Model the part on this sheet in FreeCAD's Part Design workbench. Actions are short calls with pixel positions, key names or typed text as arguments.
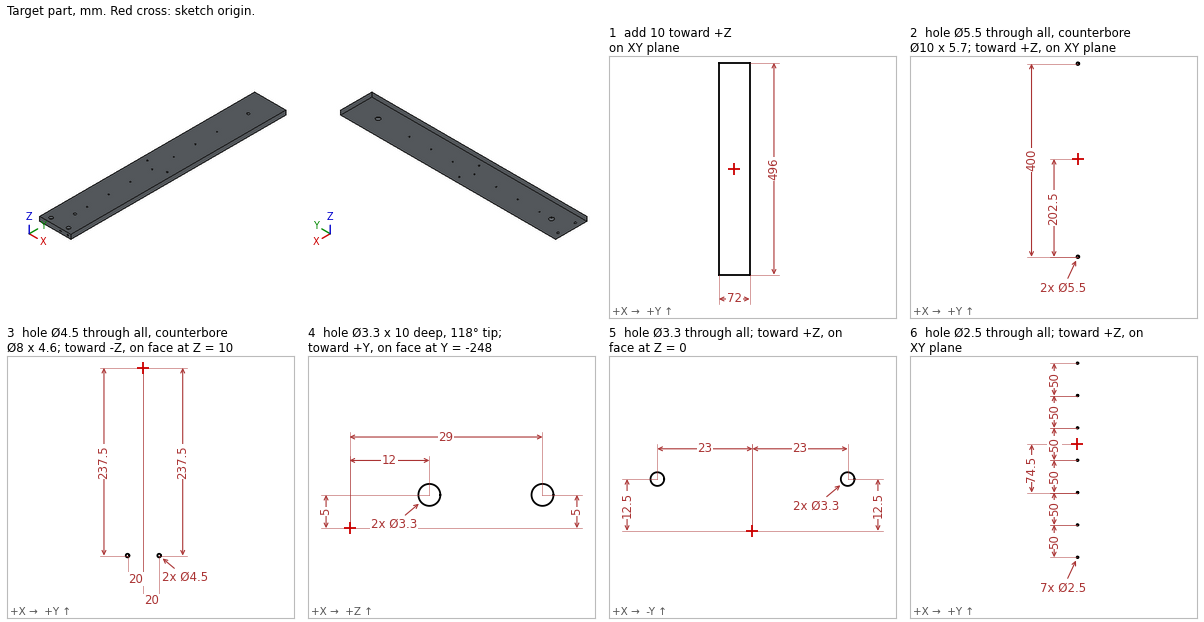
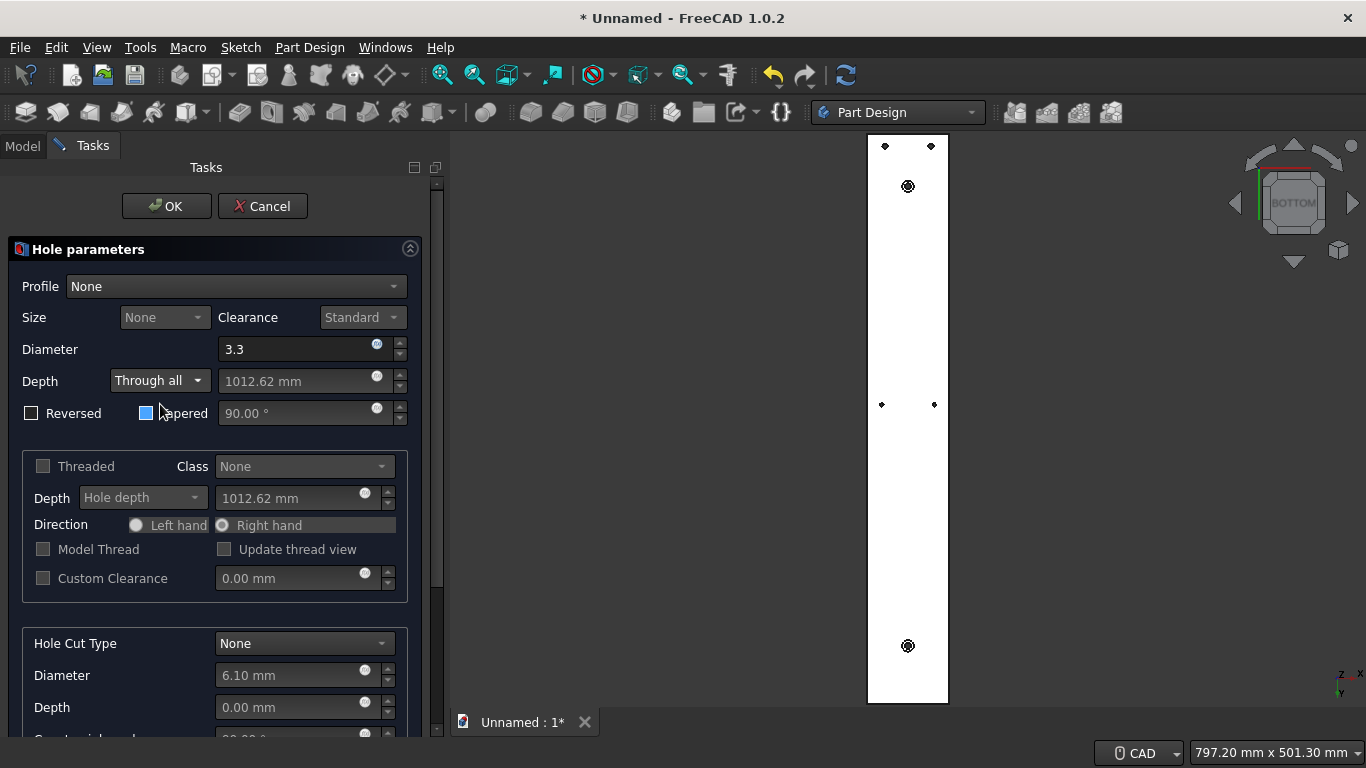
click(167, 206)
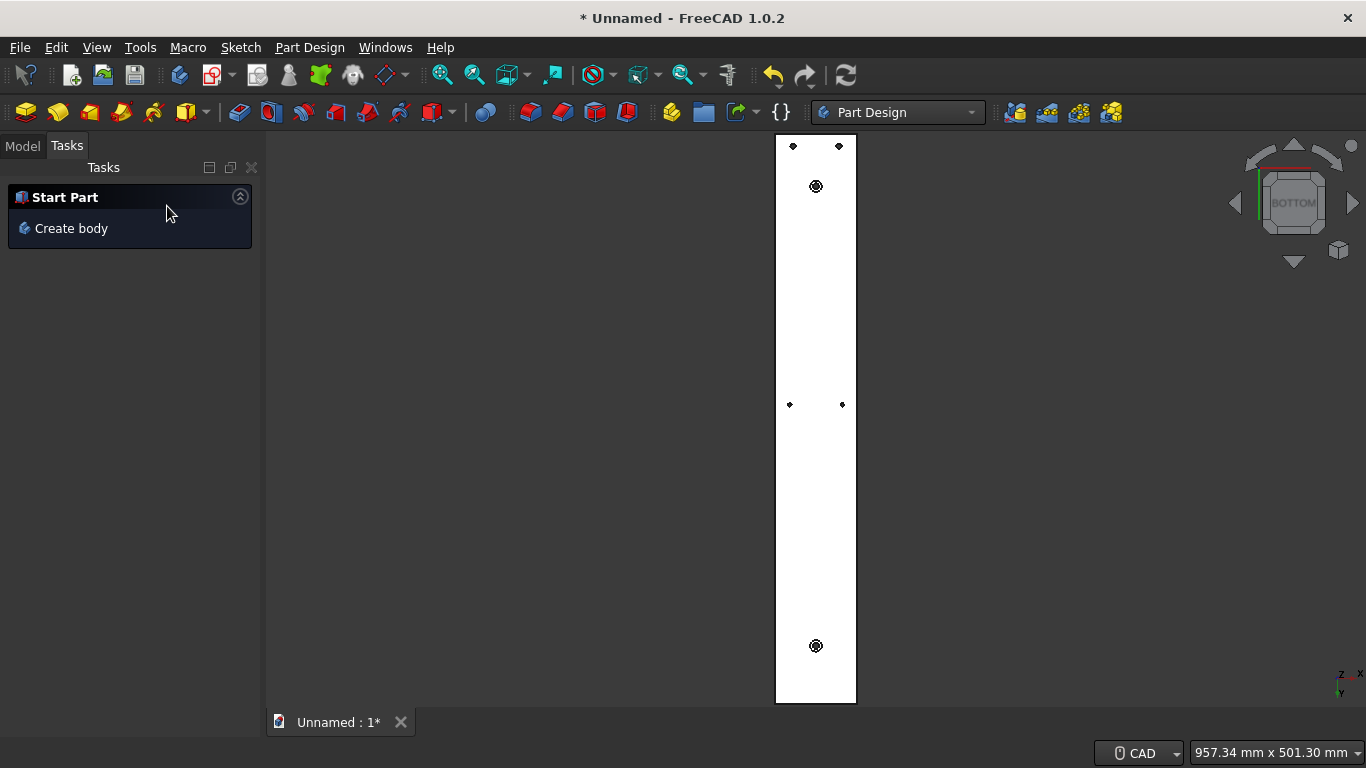
click(212, 76)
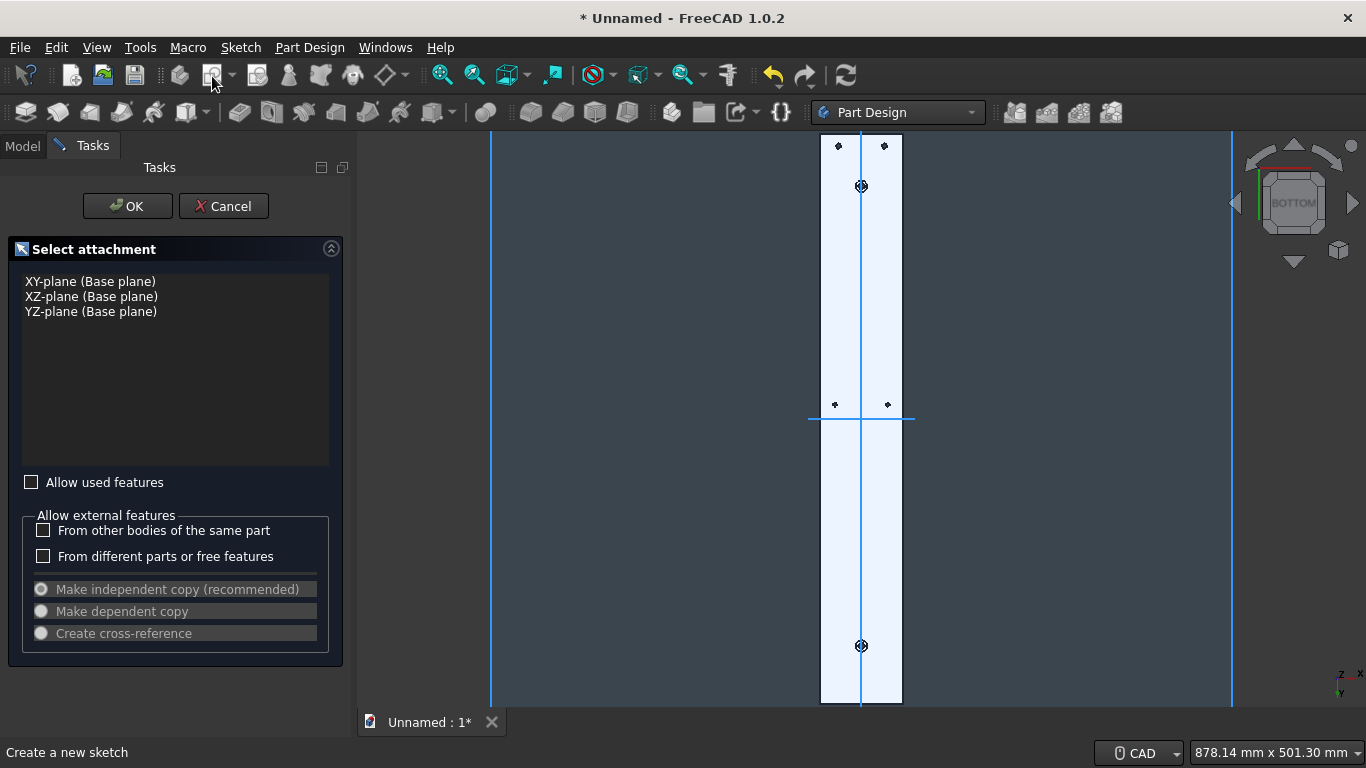
click(82, 282)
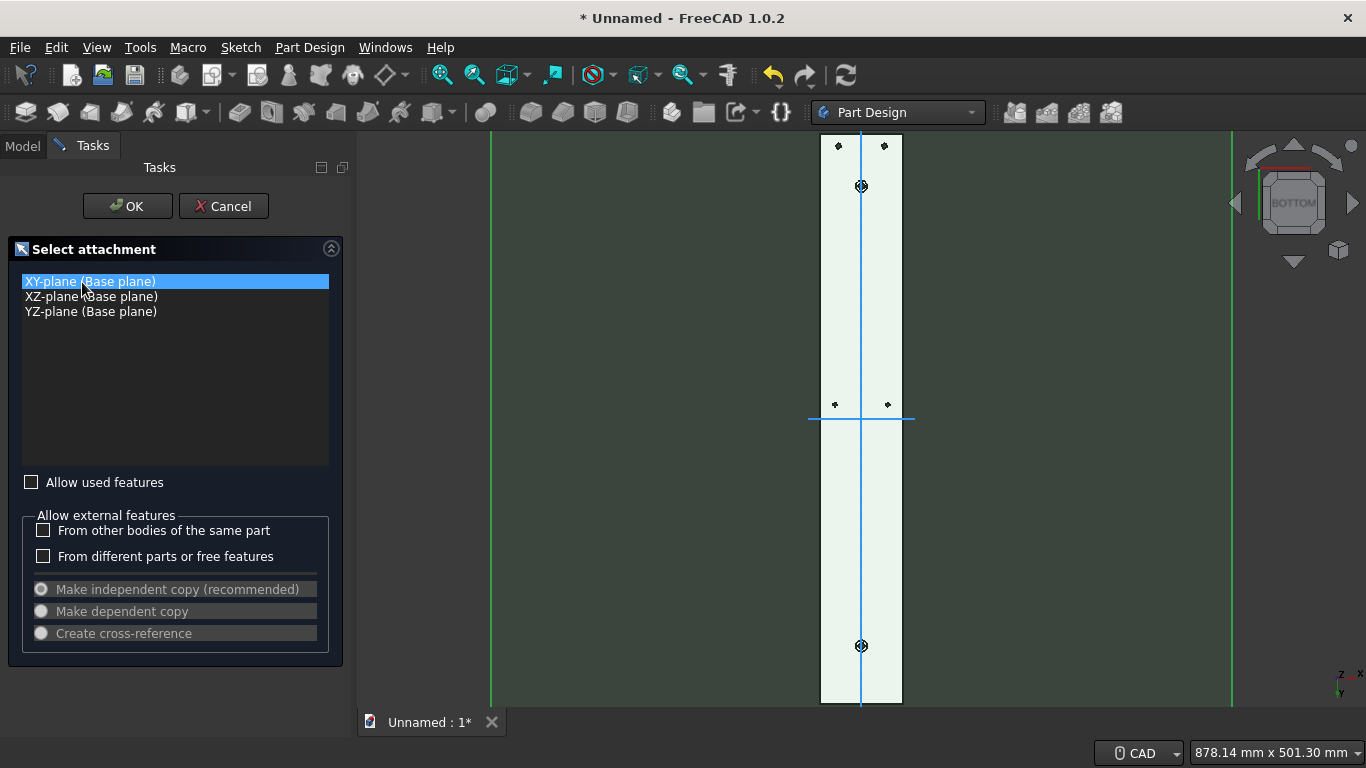
click(128, 206)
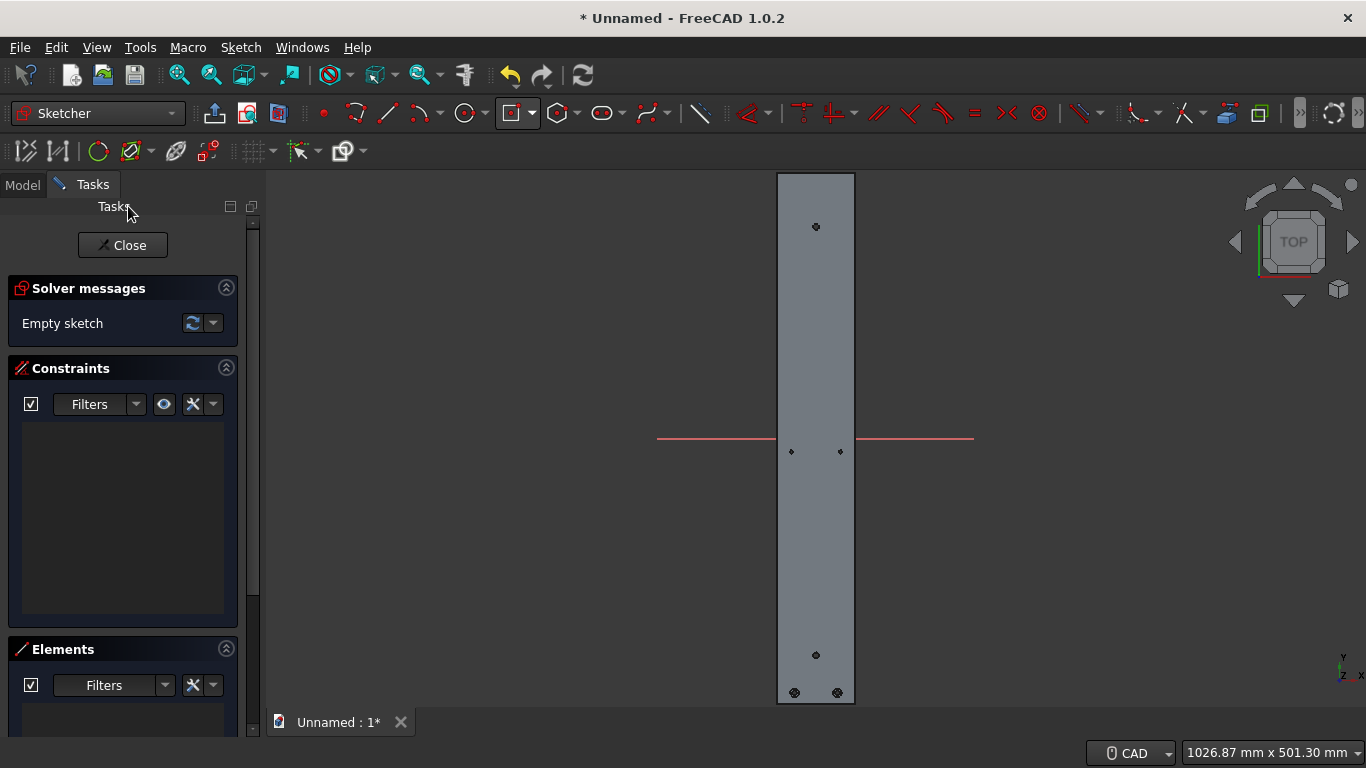
click(280, 114)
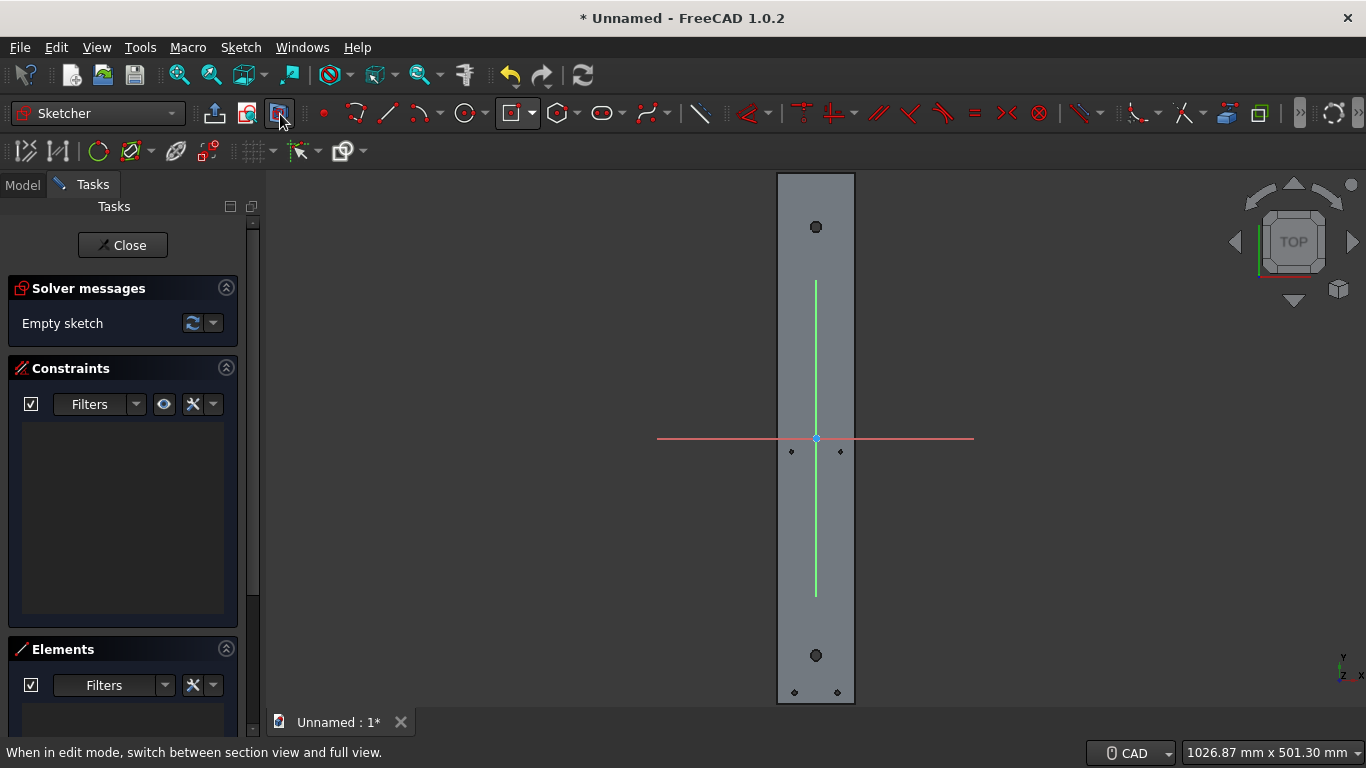
click(466, 114)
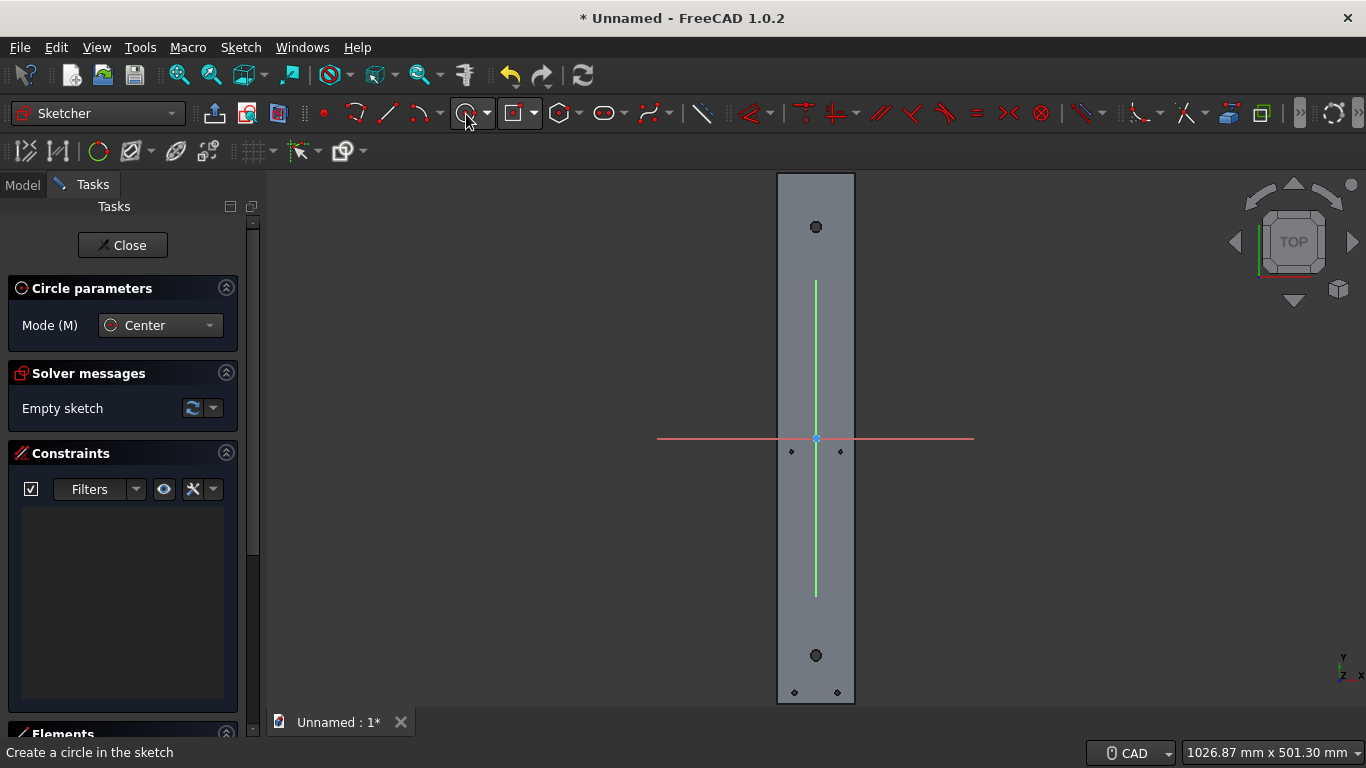
scroll(816, 625, up, 15)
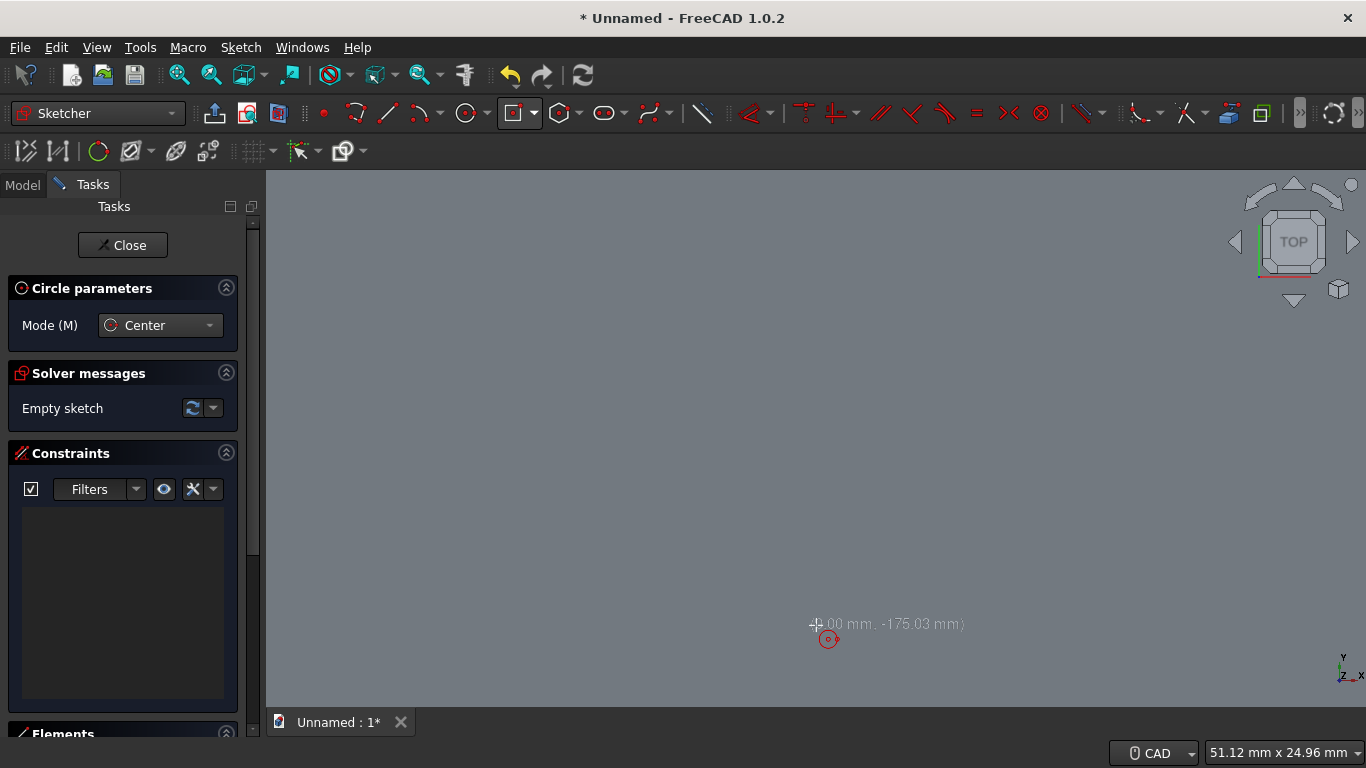
scroll(744, 598, down, 15)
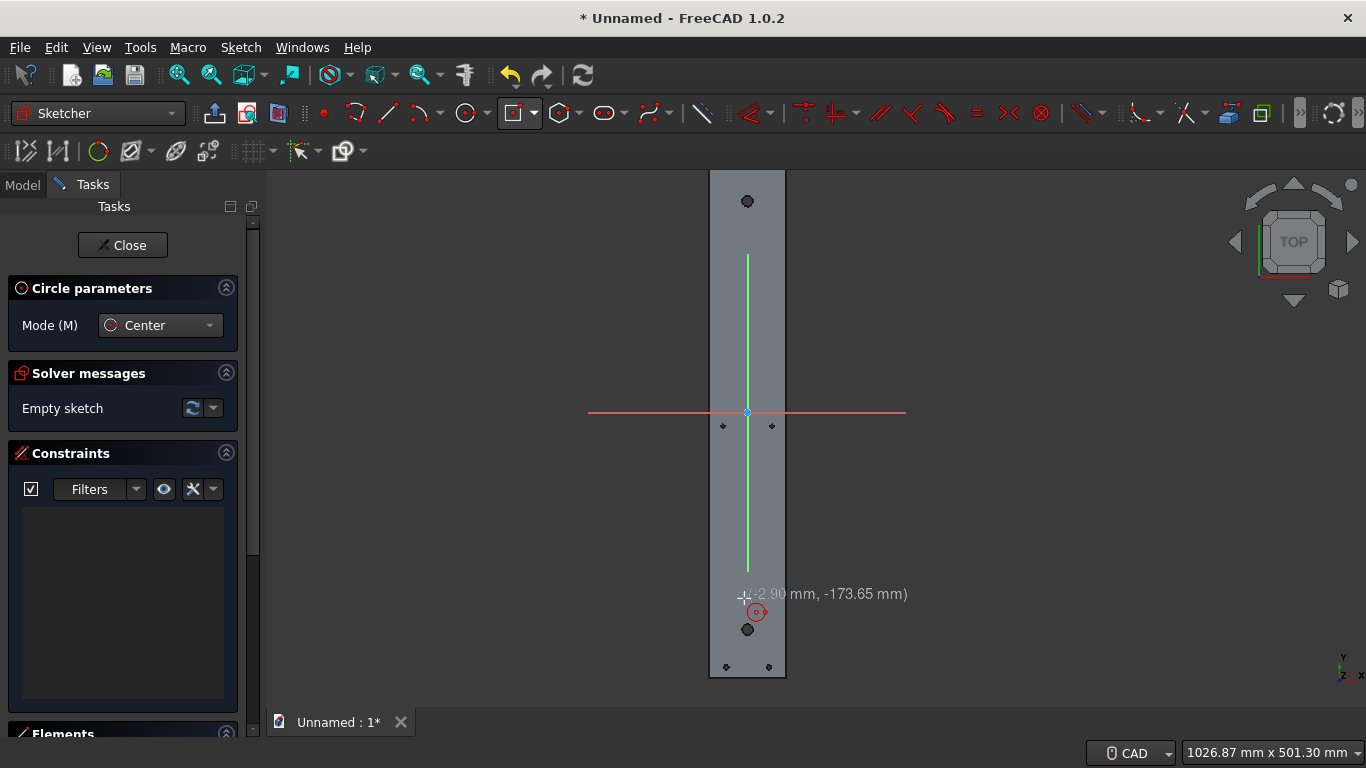
click(748, 600)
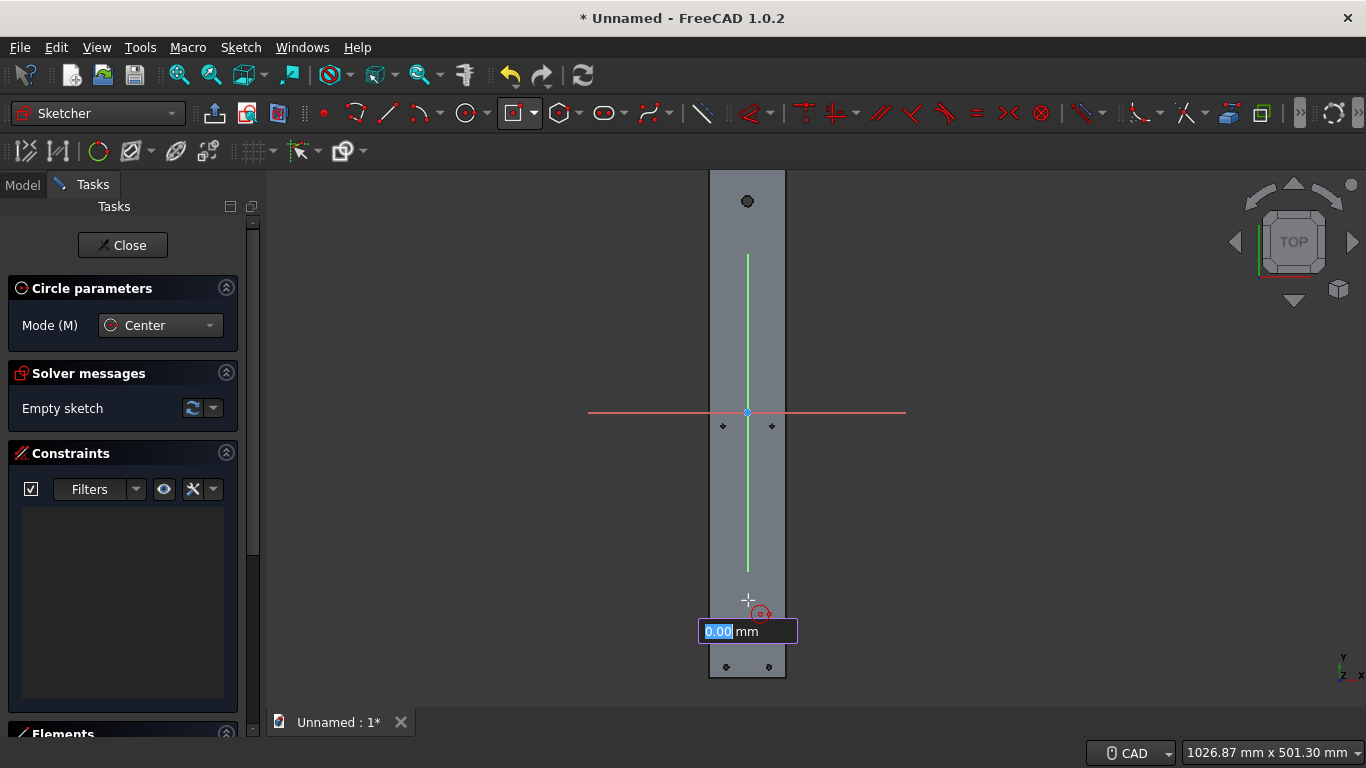
scroll(749, 599, up, 13)